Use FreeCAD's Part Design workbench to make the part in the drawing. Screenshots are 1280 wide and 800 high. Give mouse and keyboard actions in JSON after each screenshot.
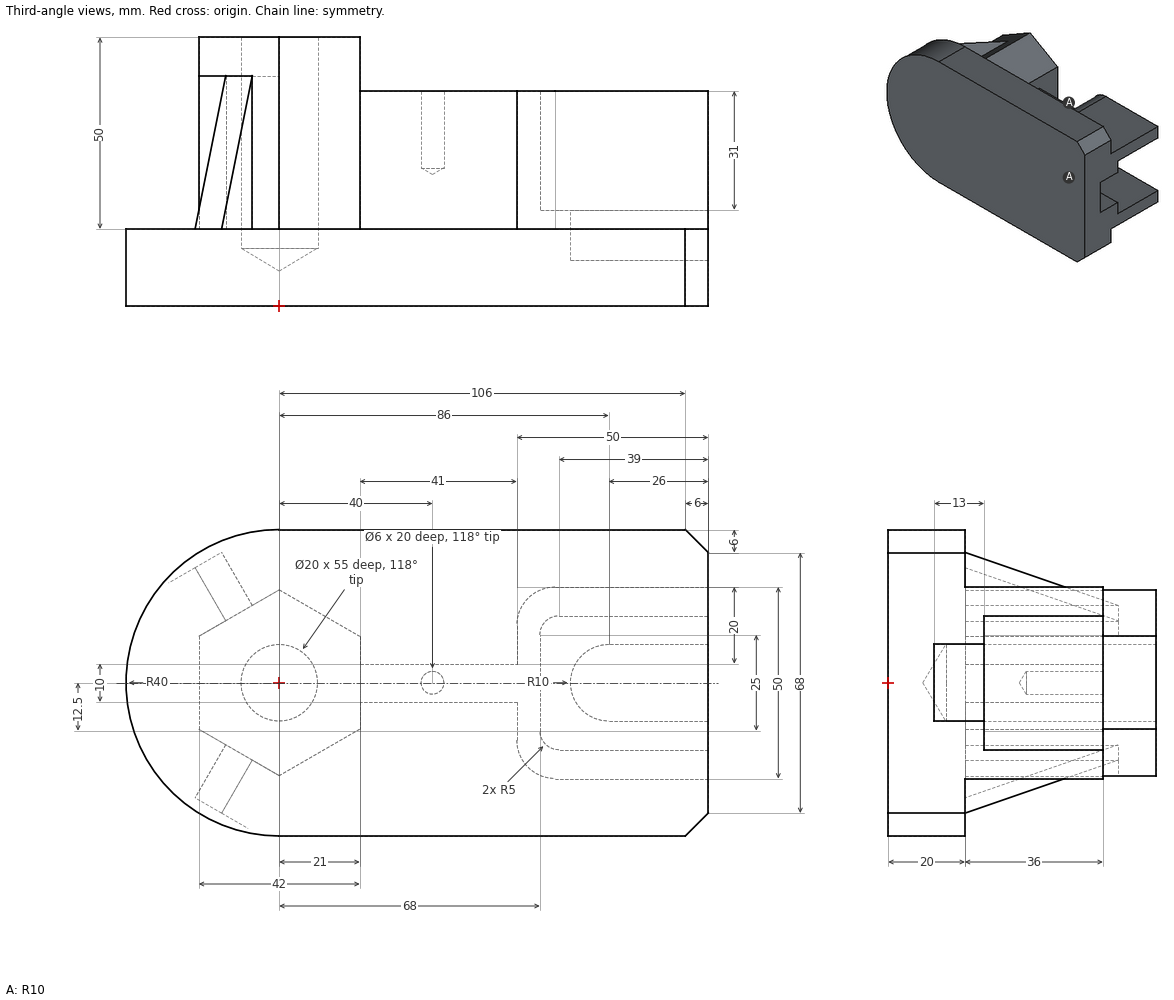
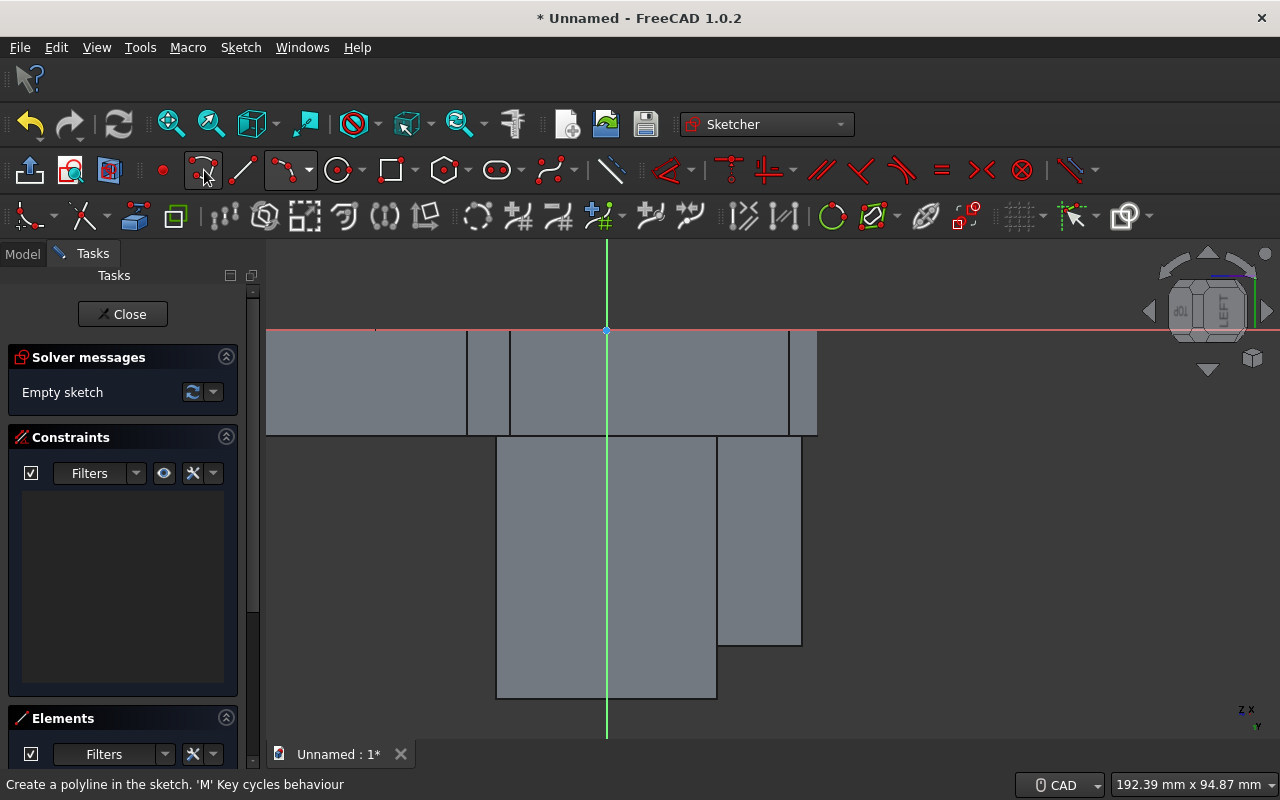
{"action": "left_click", "coordinate": [802, 436]}
{"action": "left_click", "coordinate": [717, 646]}
{"action": "left_click", "coordinate": [802, 646]}
{"action": "left_click", "coordinate": [802, 437]}
{"action": "key", "text": "Escape"}
{"action": "key", "text": "Escape"}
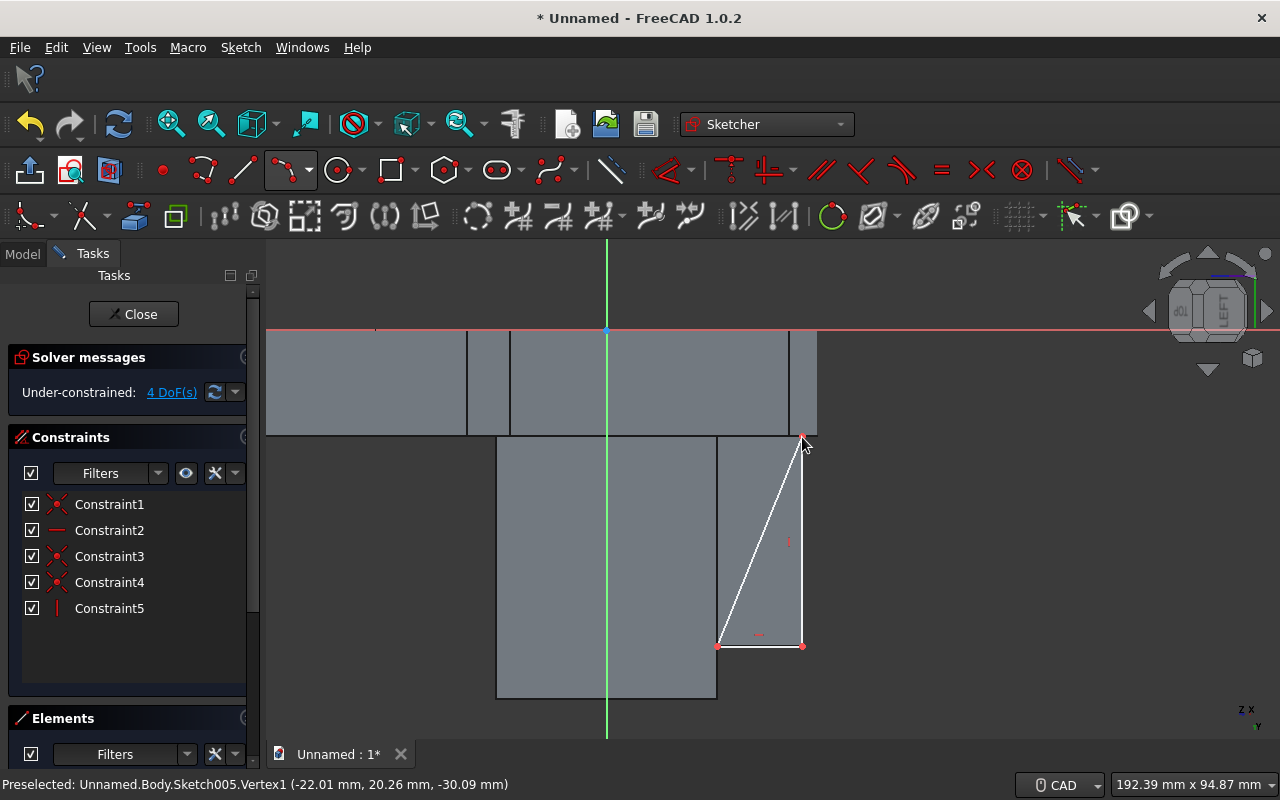
{"action": "left_click", "coordinate": [666, 170]}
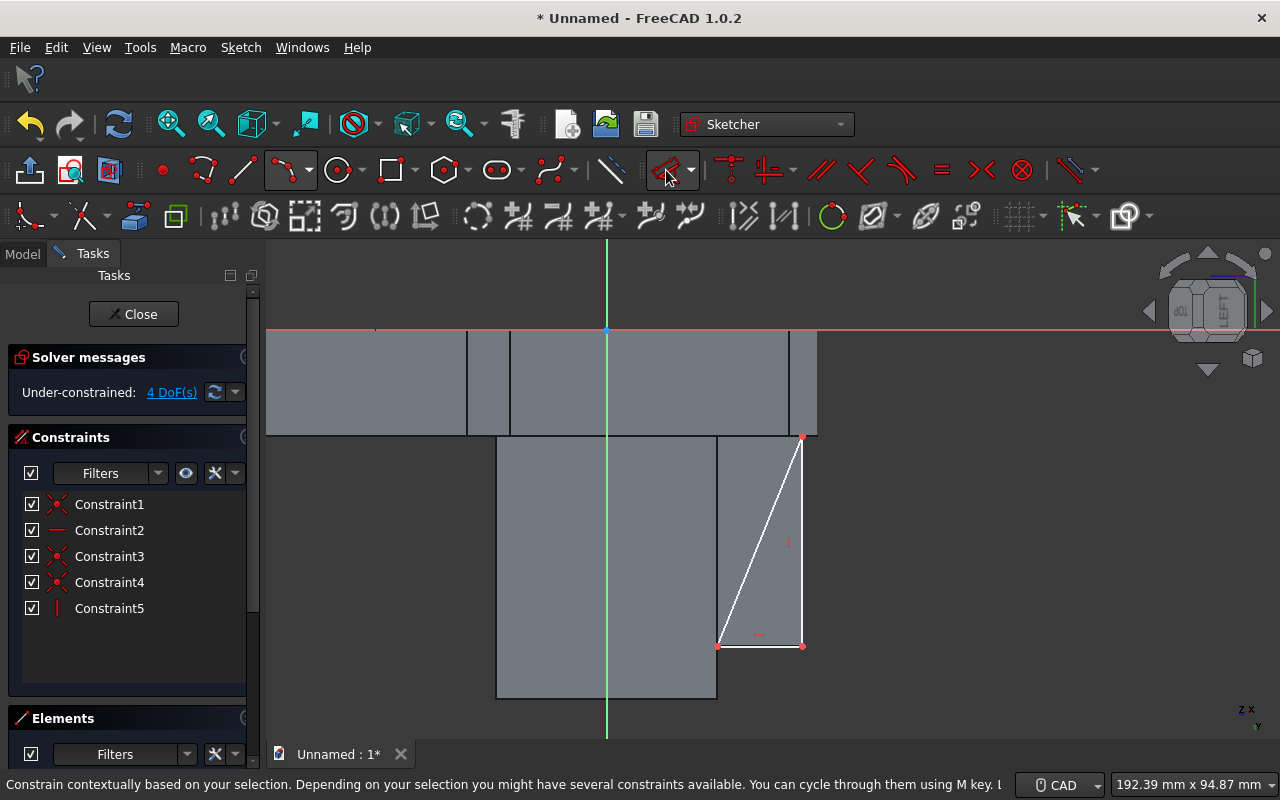
{"action": "left_click", "coordinate": [742, 647]}
{"action": "left_click", "coordinate": [760, 681]}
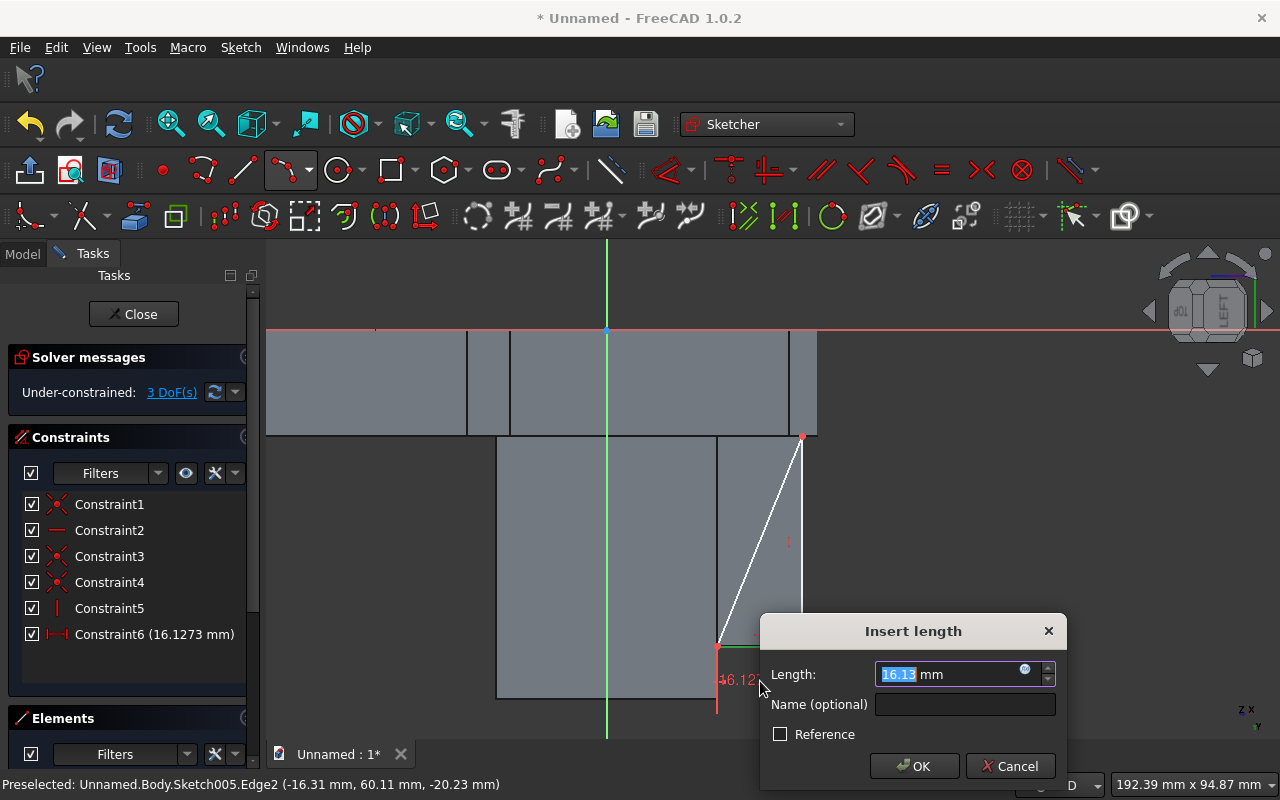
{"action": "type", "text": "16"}
{"action": "key", "text": "Return"}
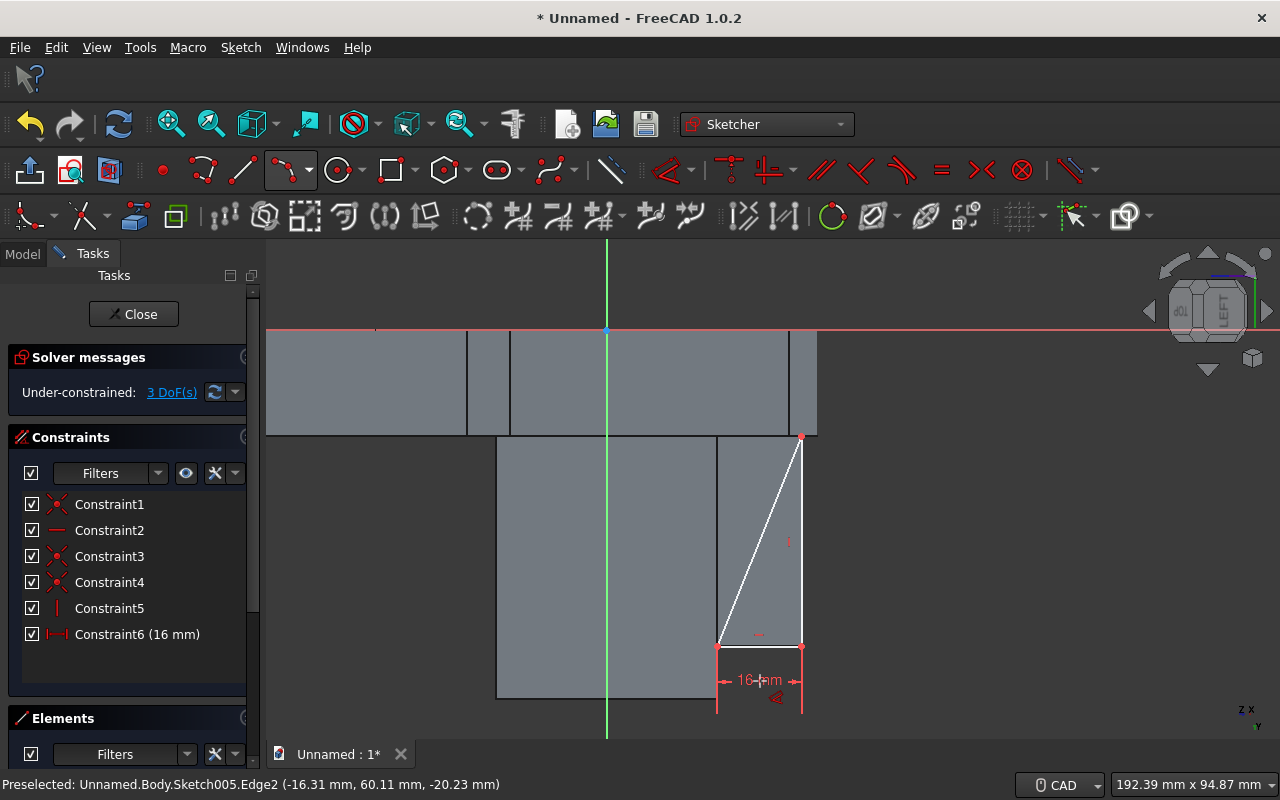
{"action": "left_click", "coordinate": [802, 584]}
{"action": "left_click", "coordinate": [836, 542]}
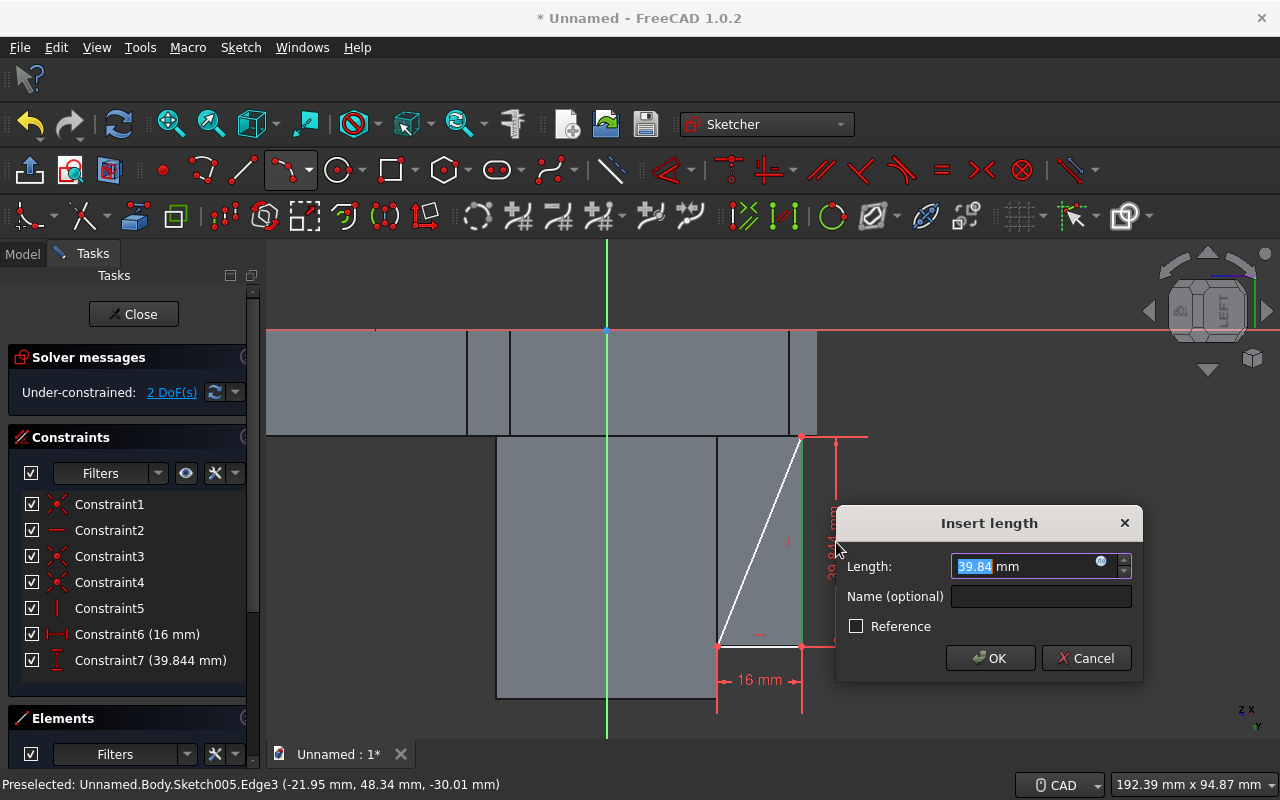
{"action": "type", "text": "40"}
{"action": "key", "text": "Return"}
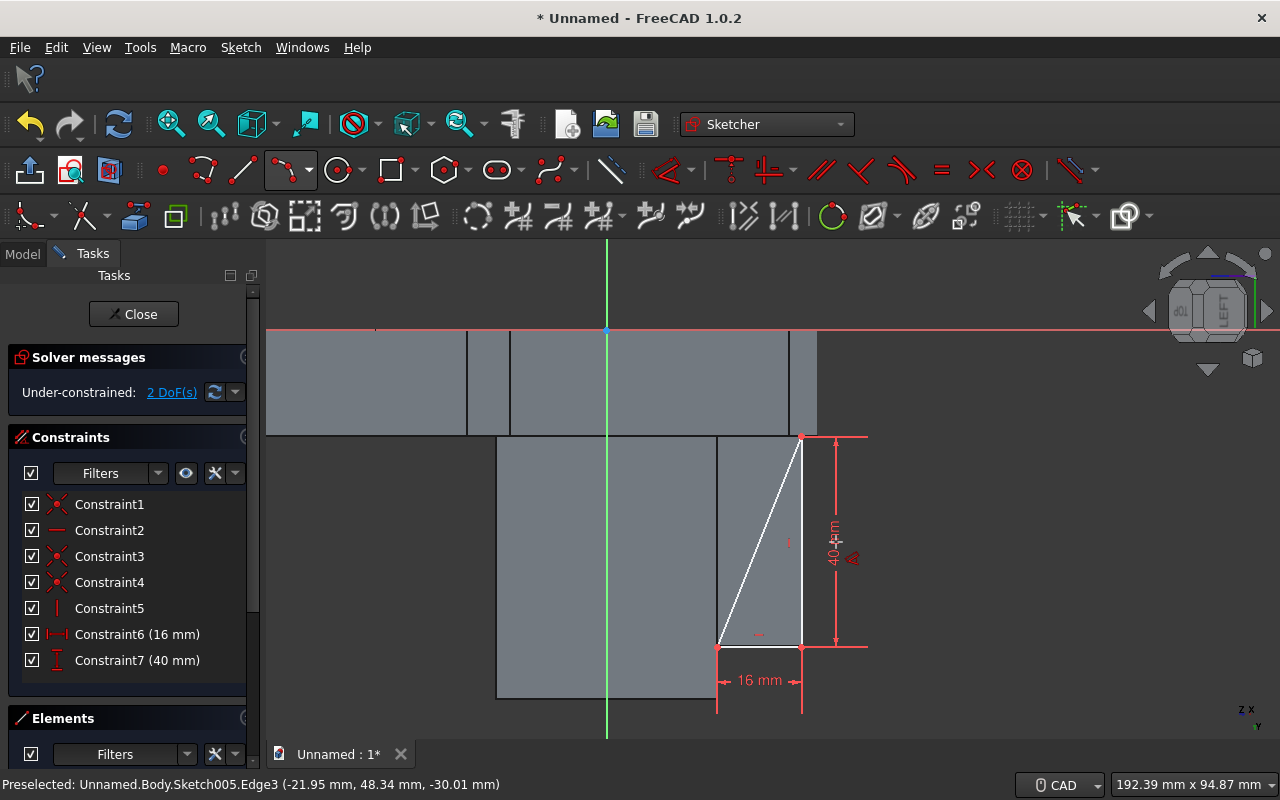
{"action": "left_click", "coordinate": [802, 437]}
{"action": "left_click", "coordinate": [704, 296]}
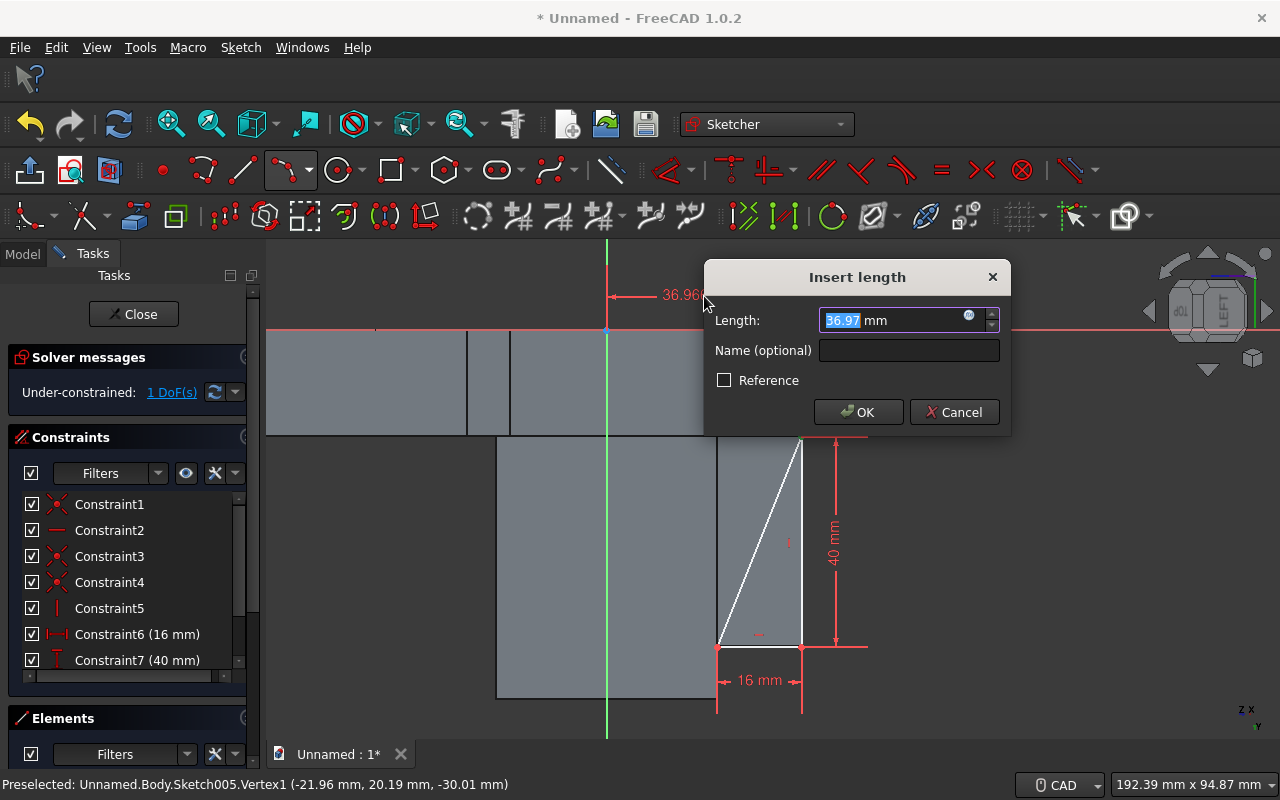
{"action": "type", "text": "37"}
{"action": "key", "text": "Return"}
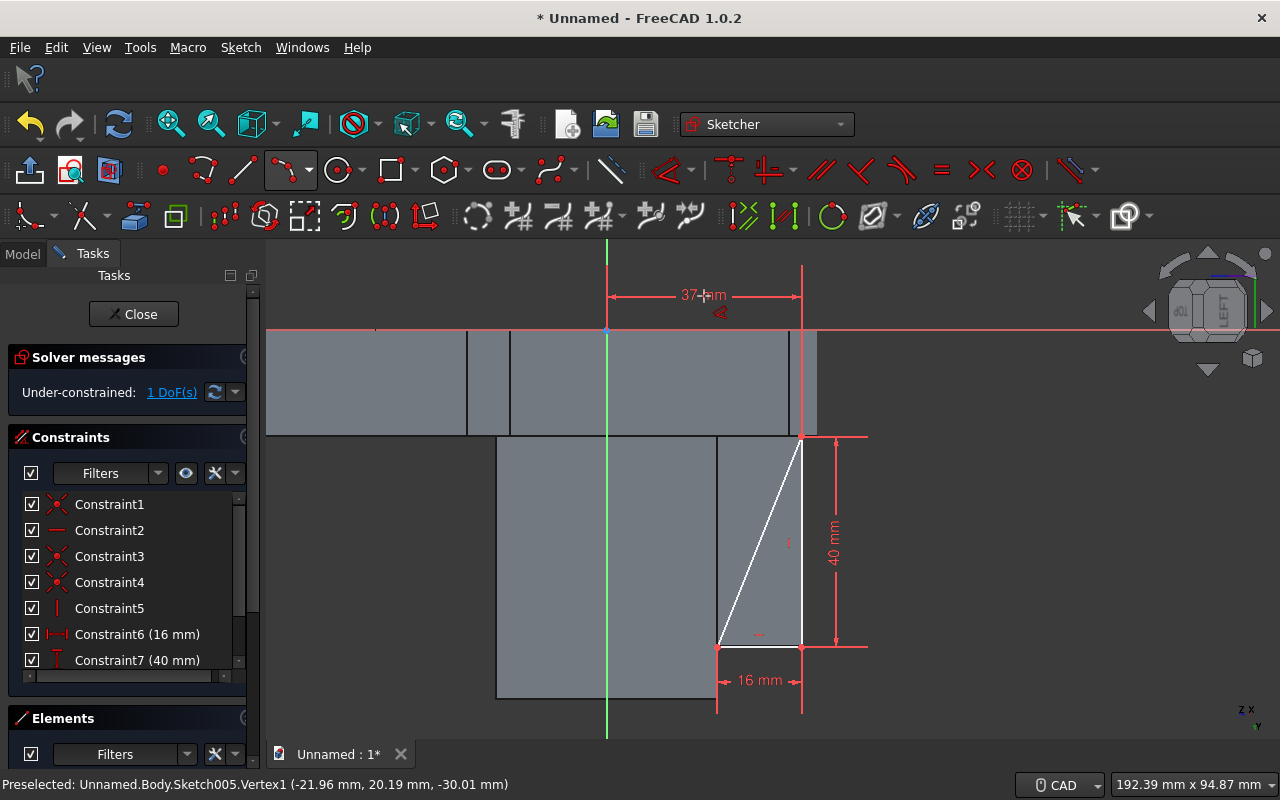
{"action": "left_click", "coordinate": [802, 437]}
{"action": "left_click", "coordinate": [573, 383]}